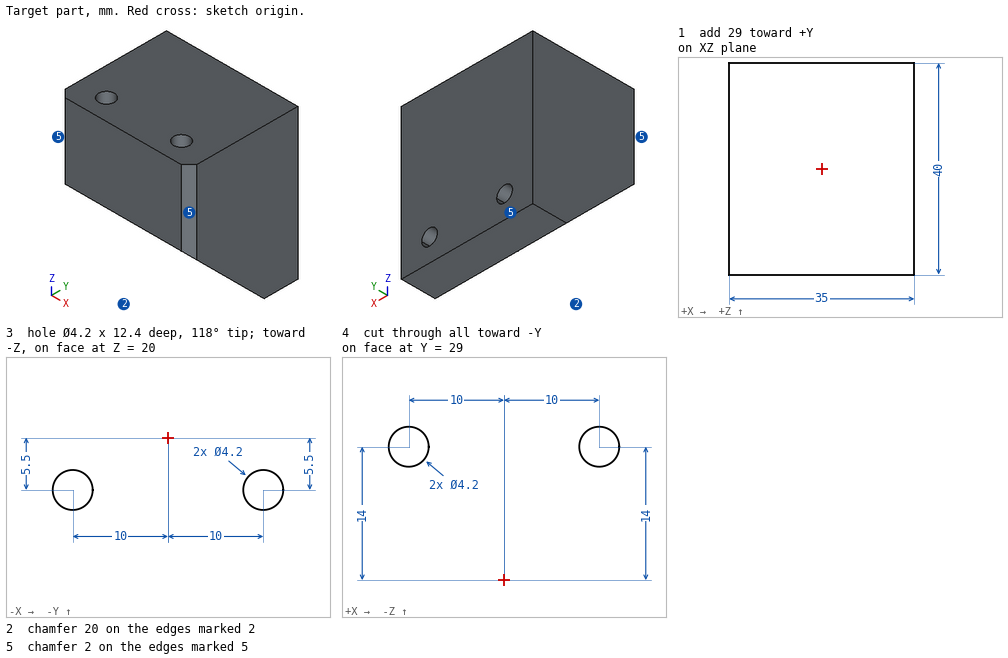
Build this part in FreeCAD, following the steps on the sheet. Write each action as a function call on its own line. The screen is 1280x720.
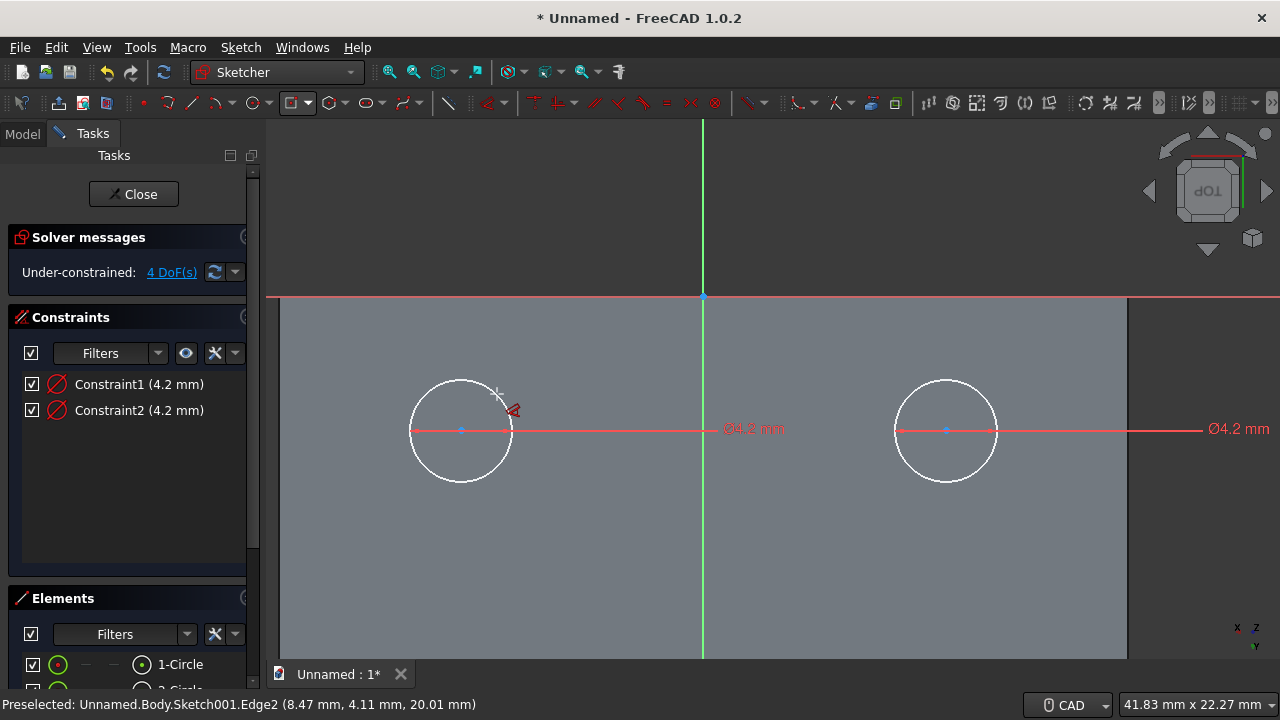
click(946, 431)
click(825, 263)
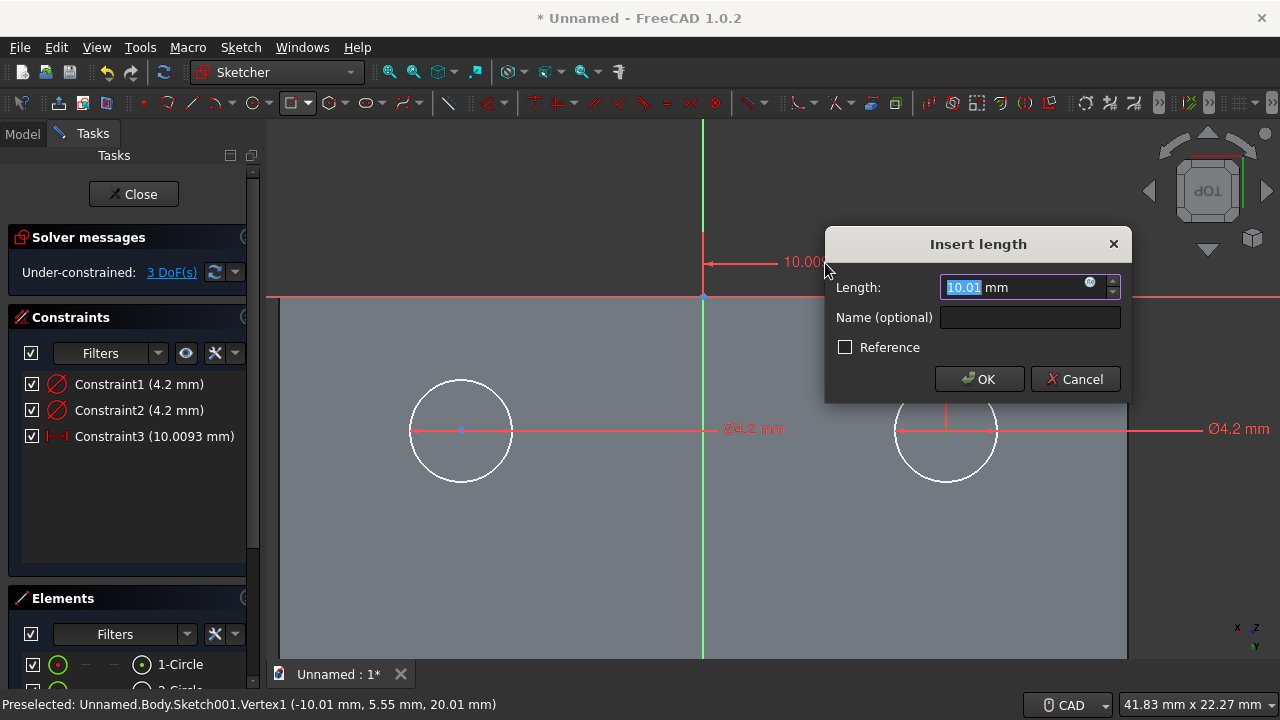
text(10)
key(Return)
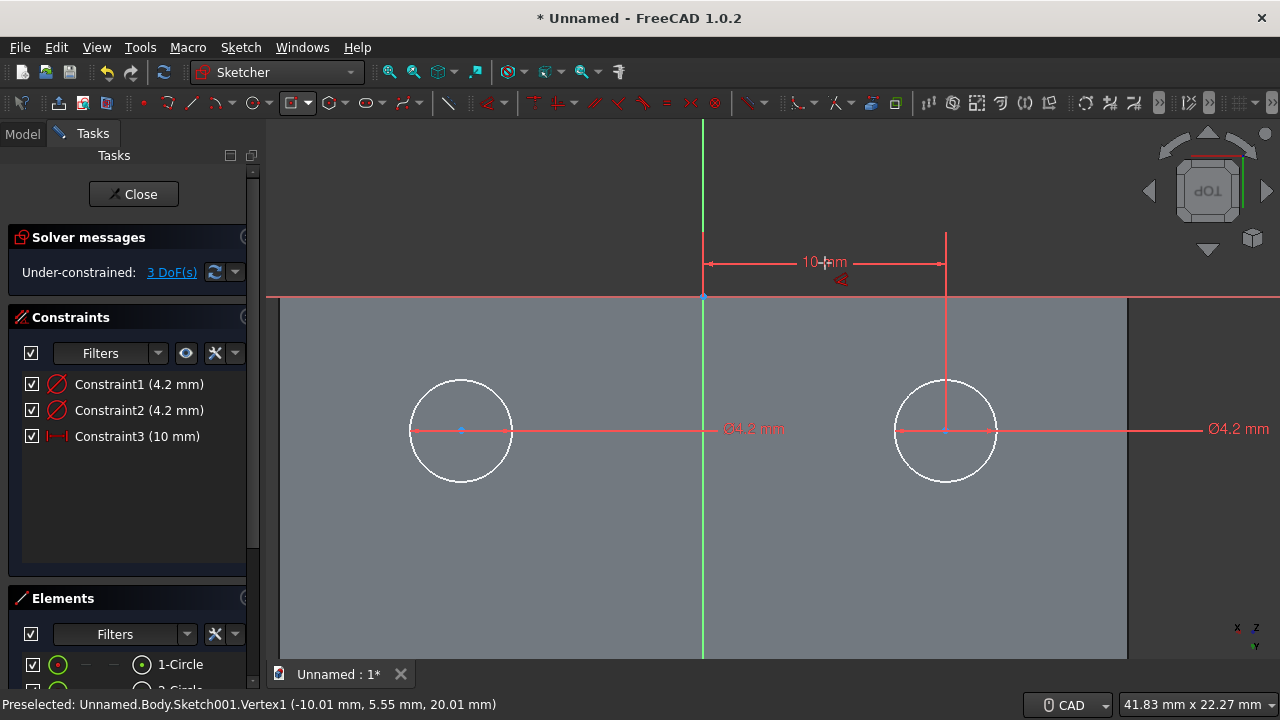
click(461, 431)
click(582, 263)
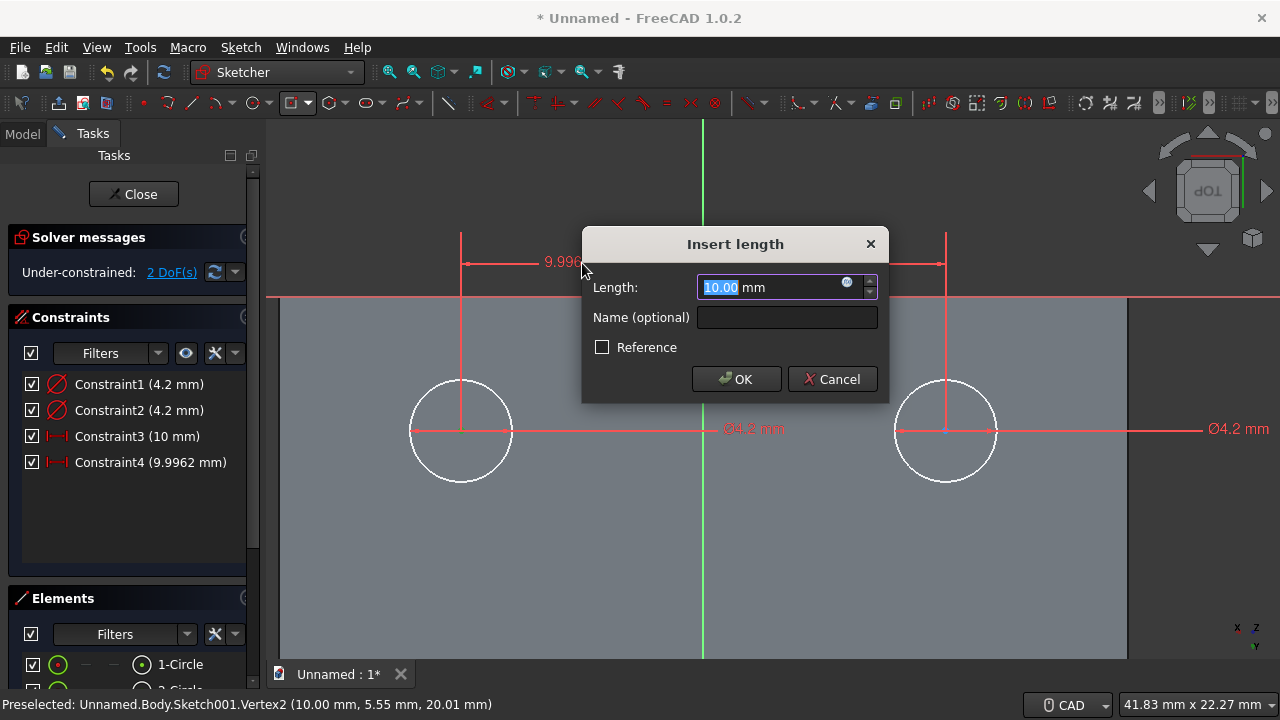
text(10)
key(Return)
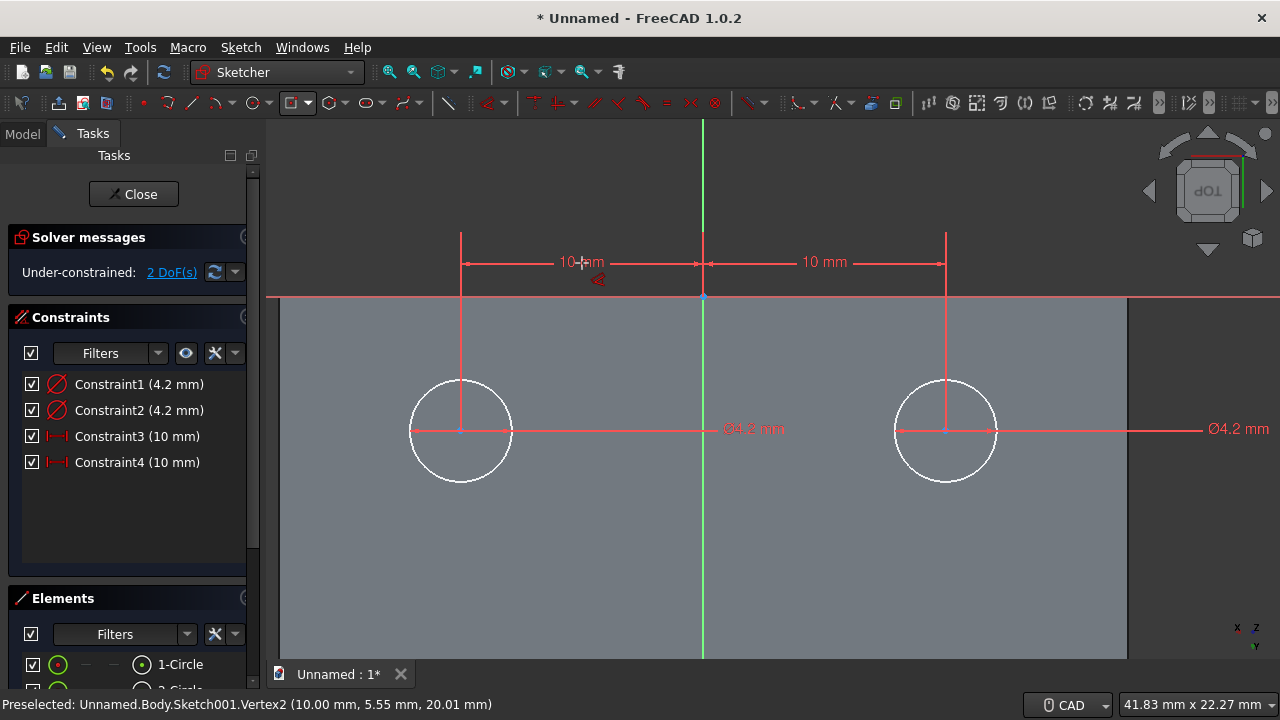
click(946, 431)
click(980, 364)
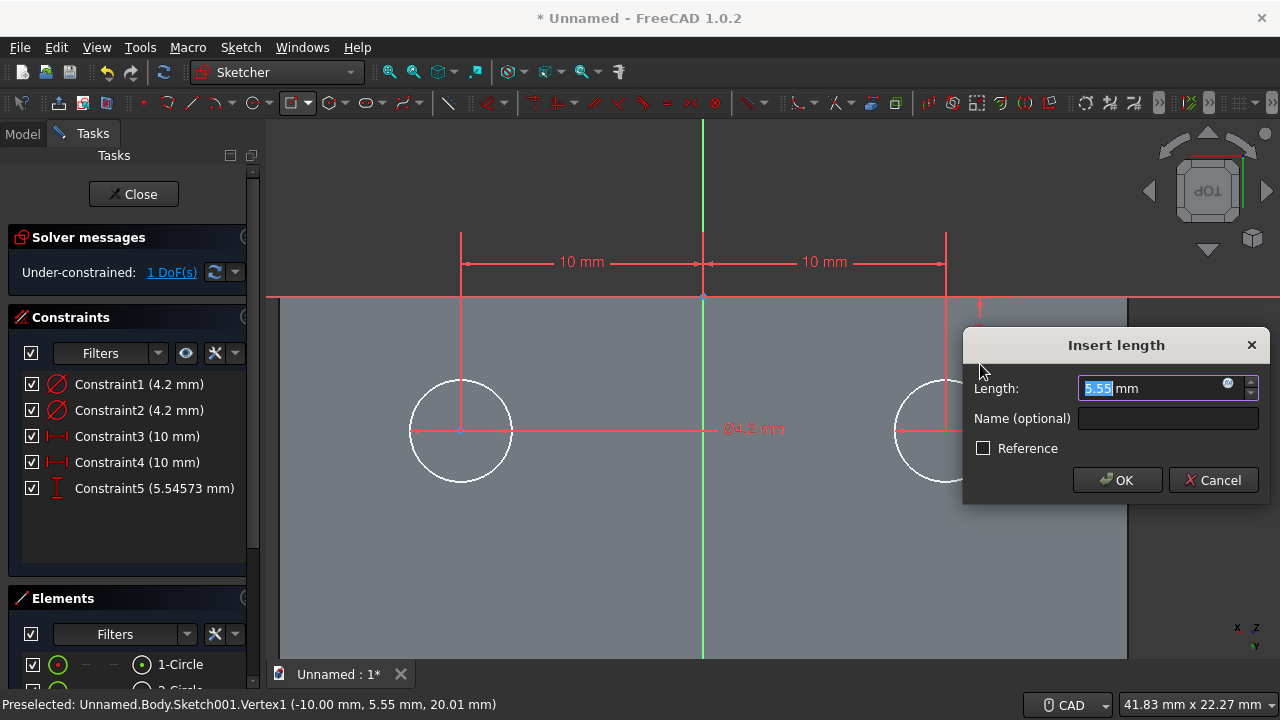
text(5.5)
key(Return)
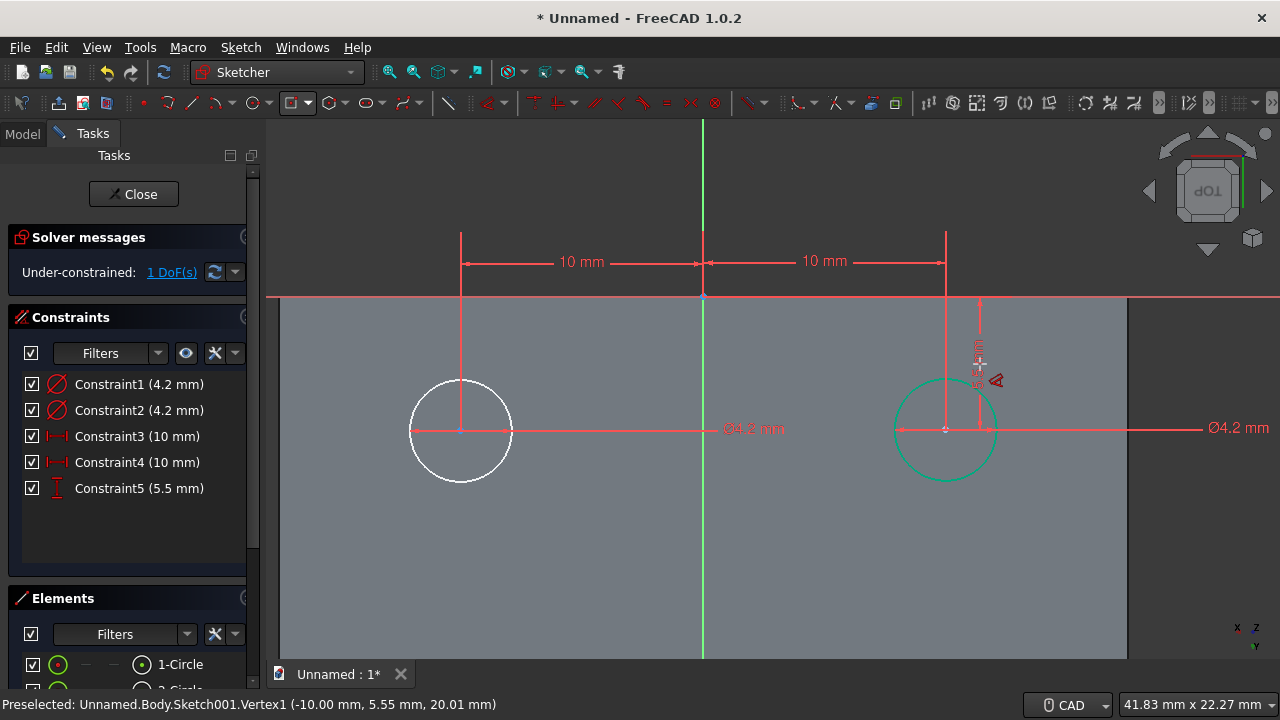
click(461, 431)
click(427, 364)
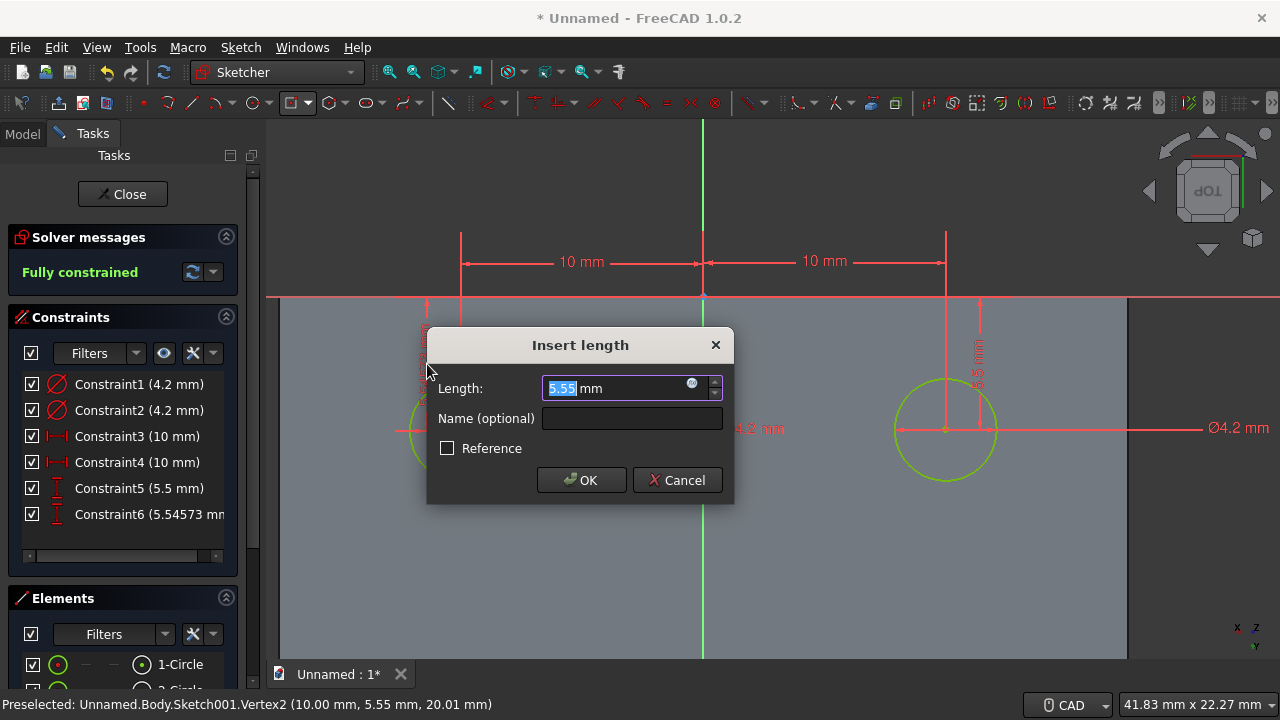
text(5.5)
key(Return)
key(Escape)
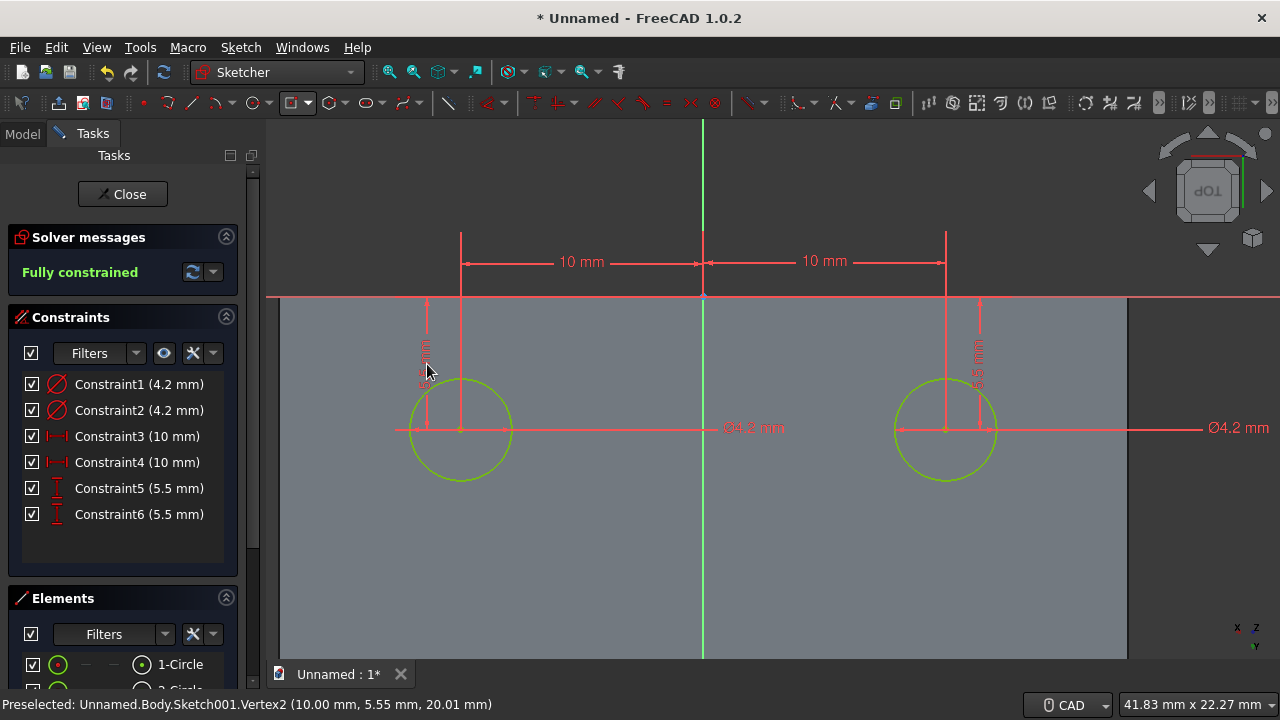
click(123, 194)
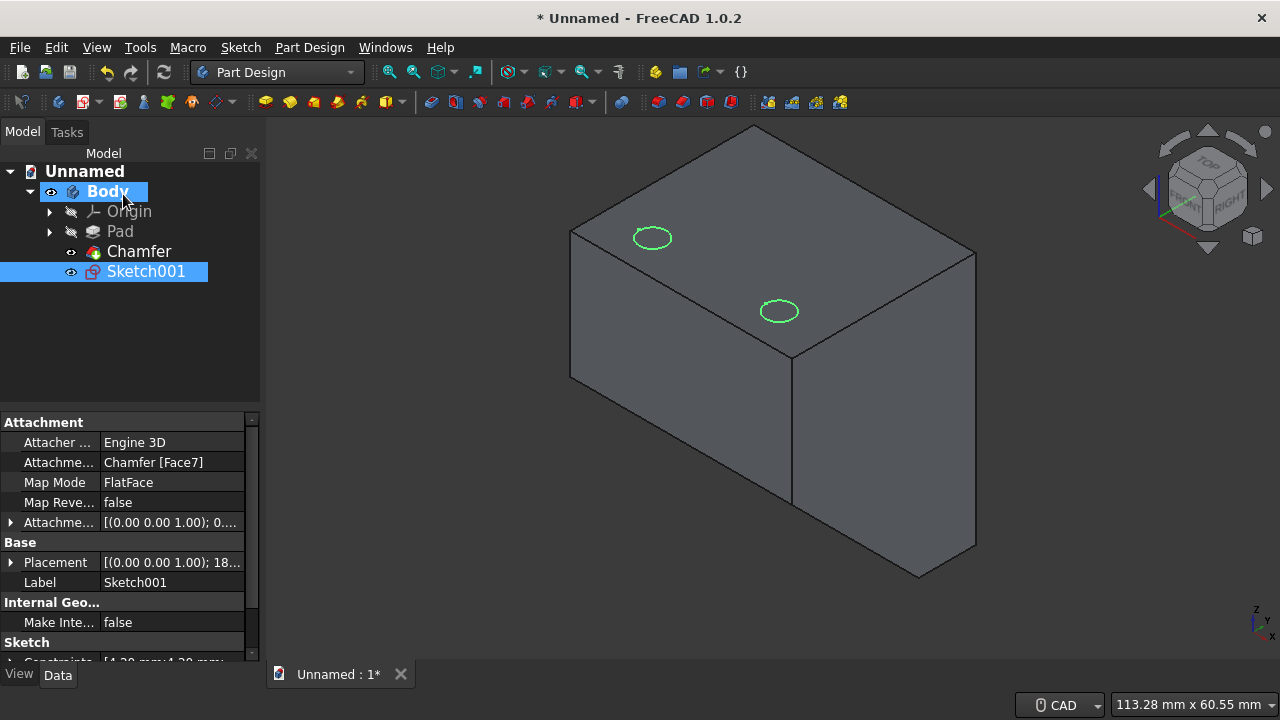
click(456, 102)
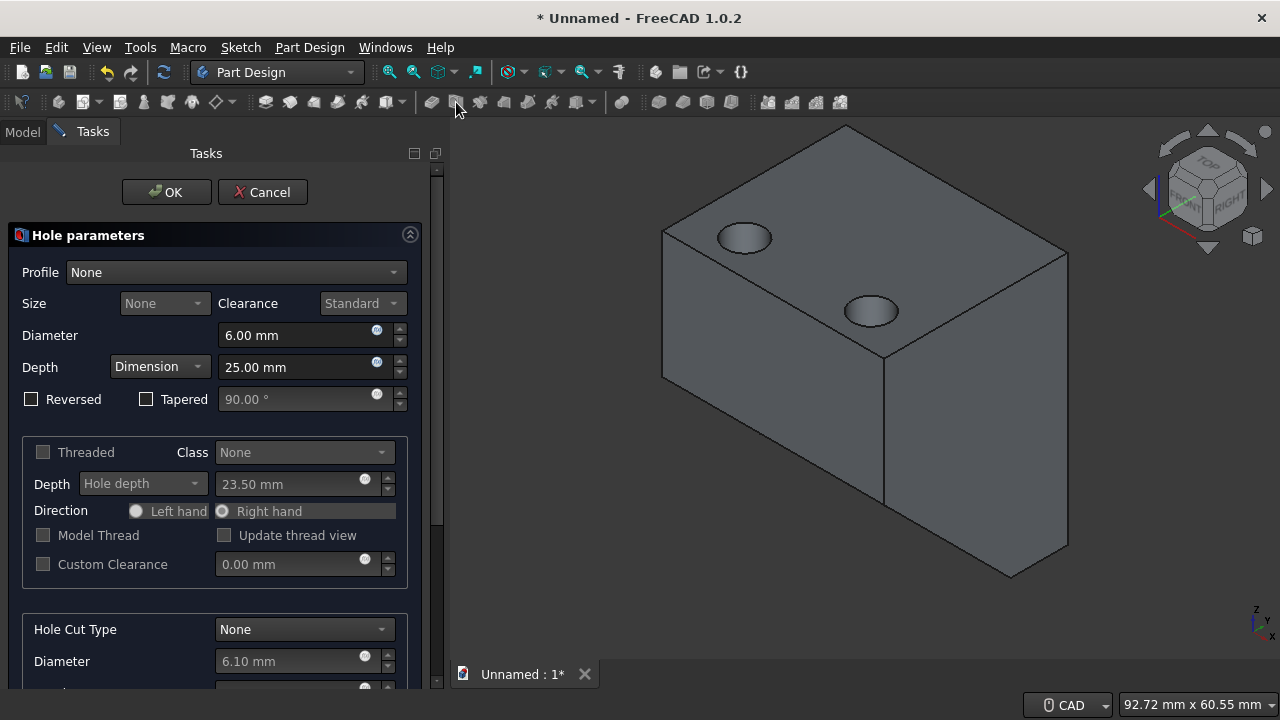
triple_click(305, 335)